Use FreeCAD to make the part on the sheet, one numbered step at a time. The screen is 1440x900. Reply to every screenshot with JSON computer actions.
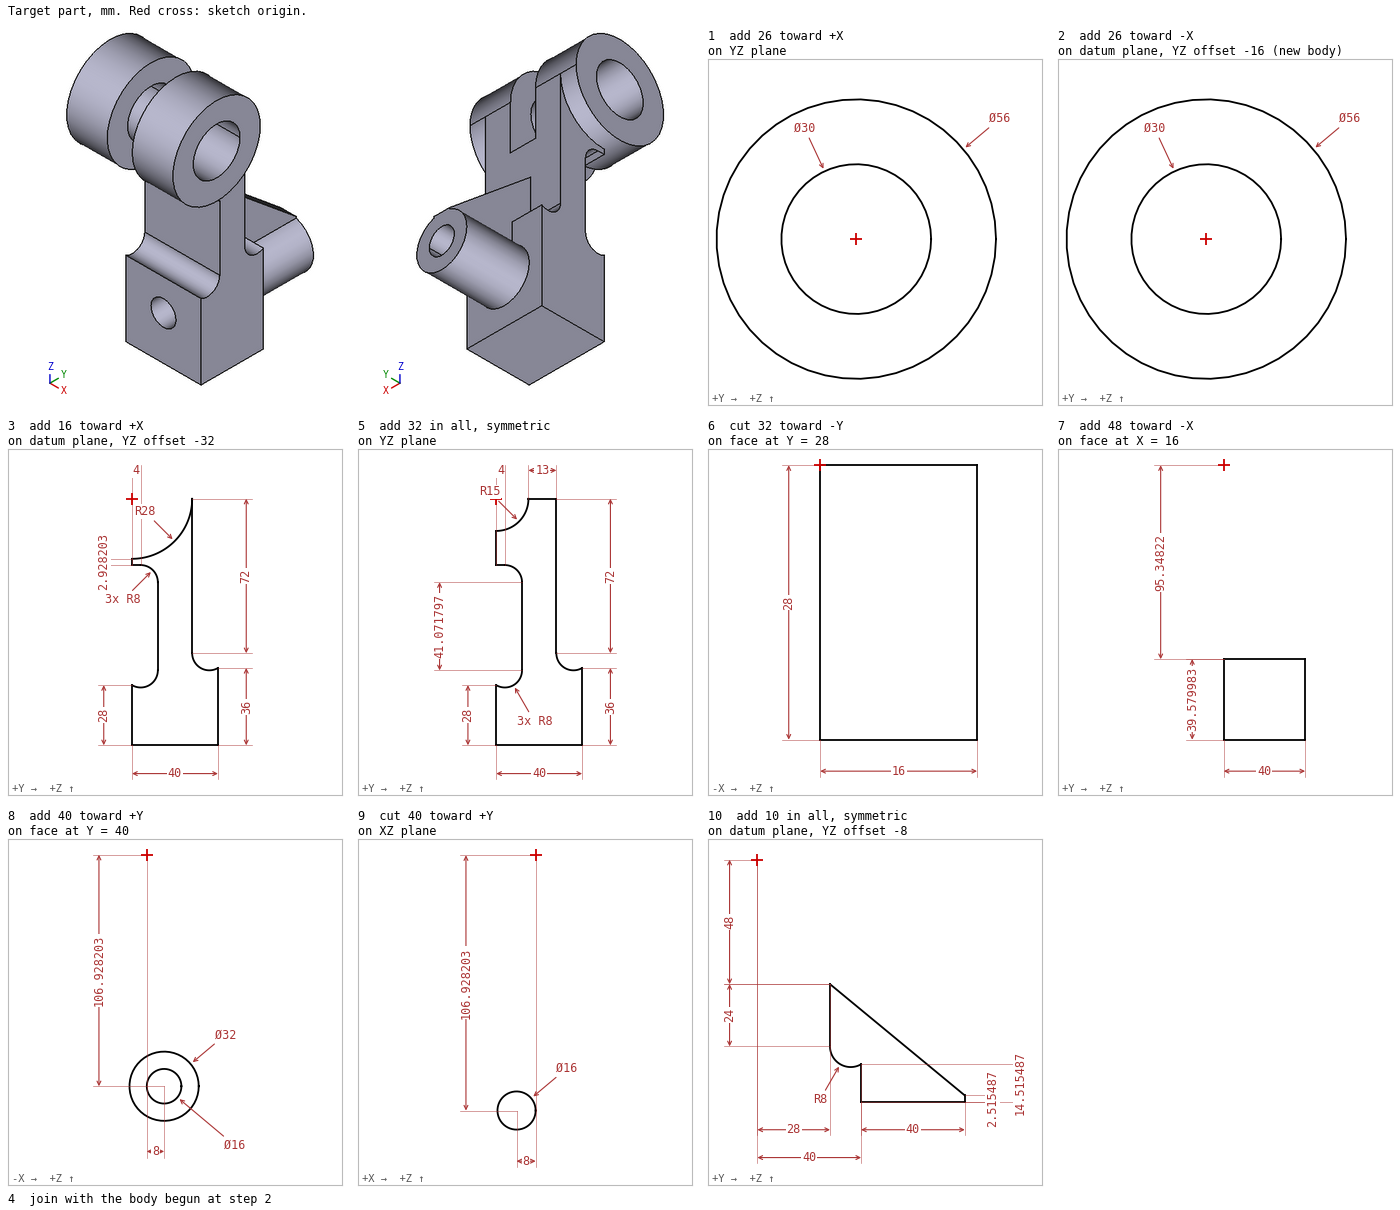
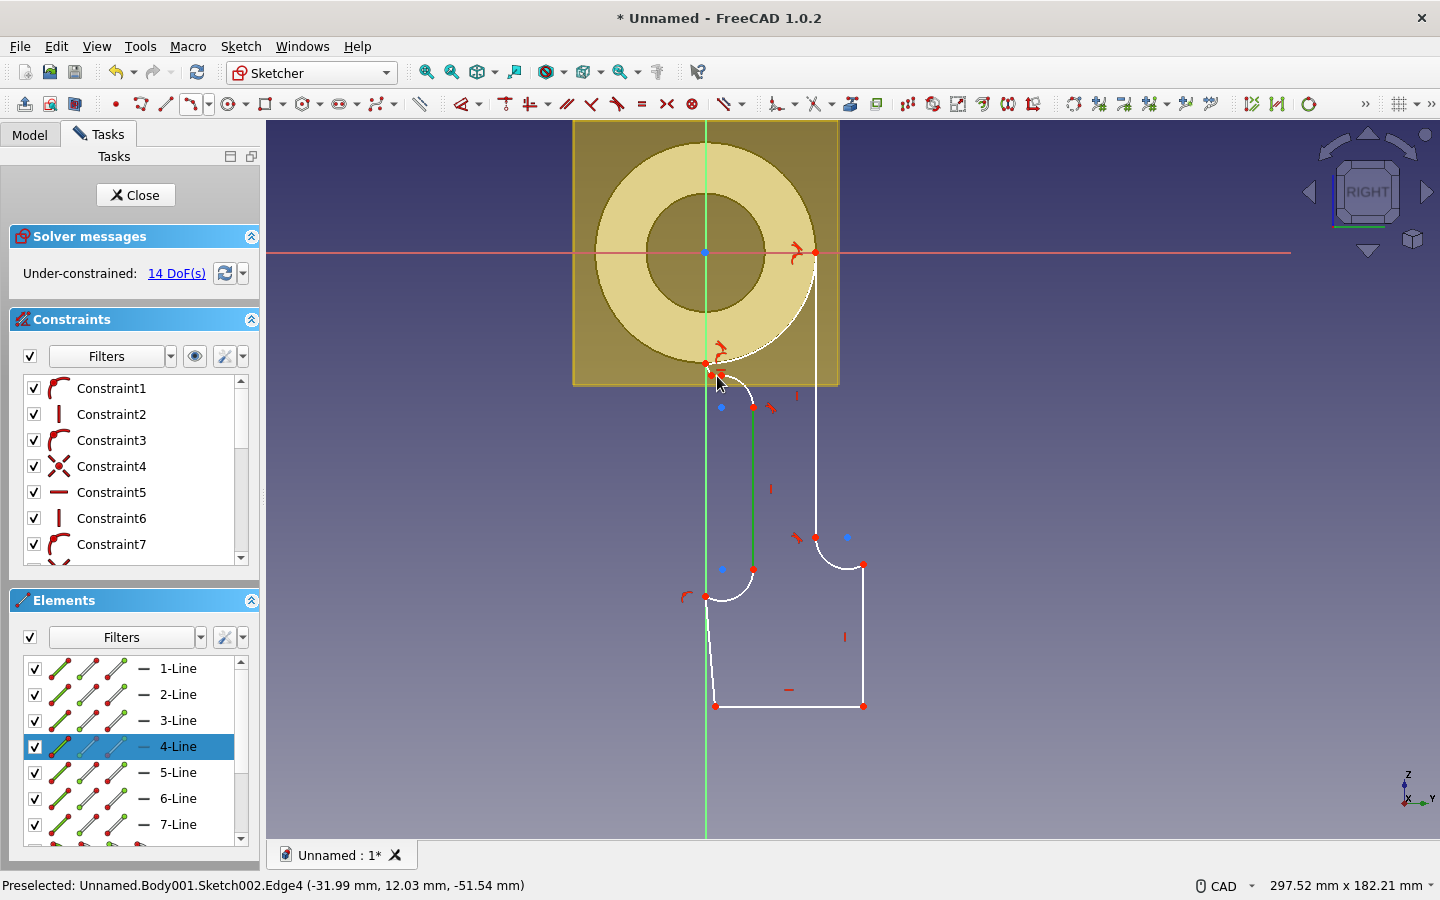
{"action": "left_click", "coordinate": [725, 601]}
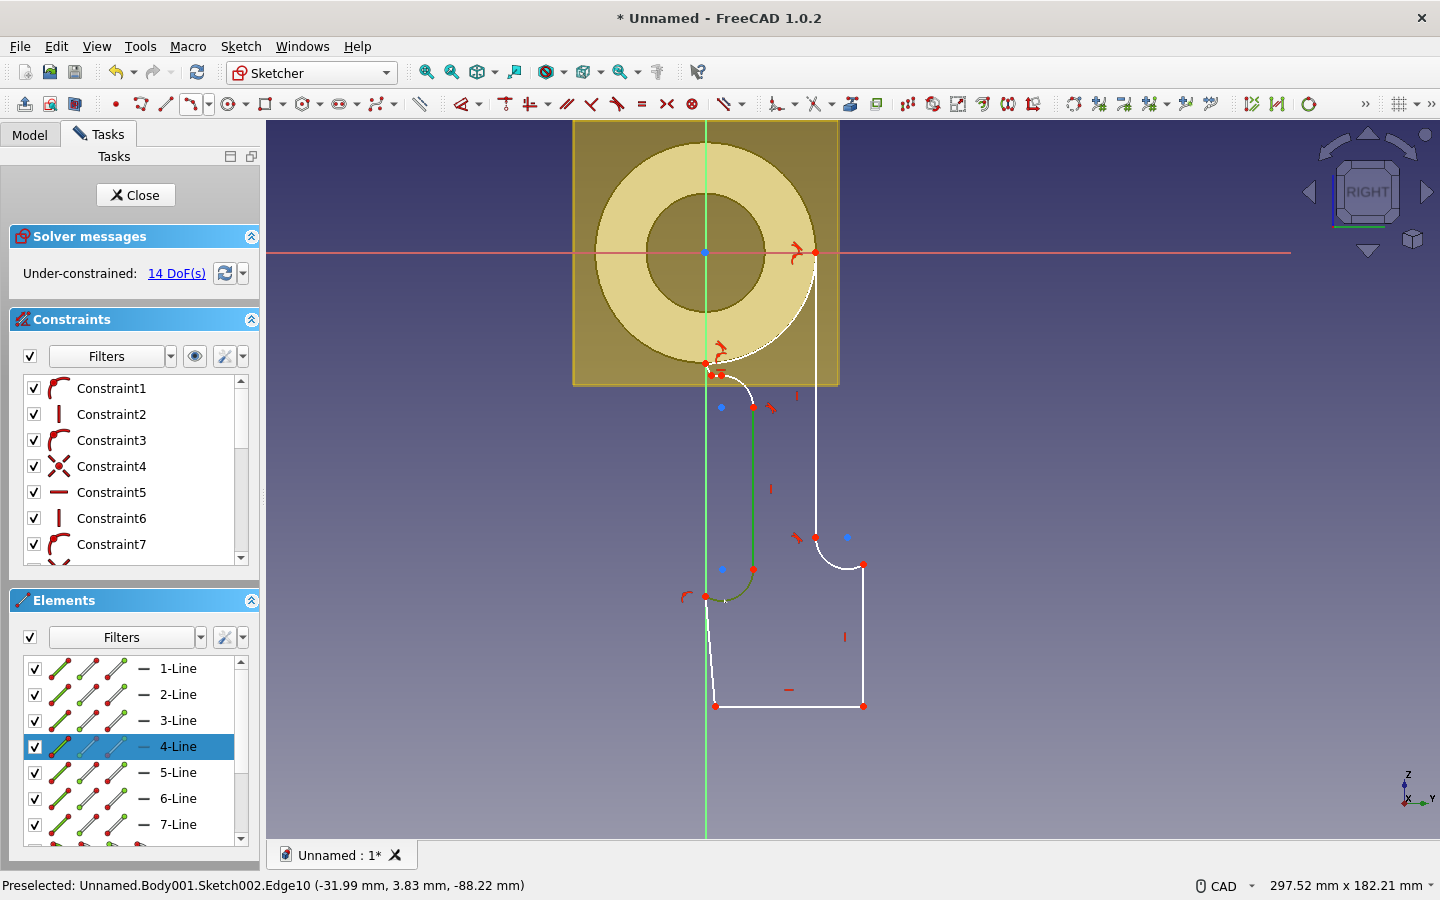
{"action": "left_click", "coordinate": [617, 104]}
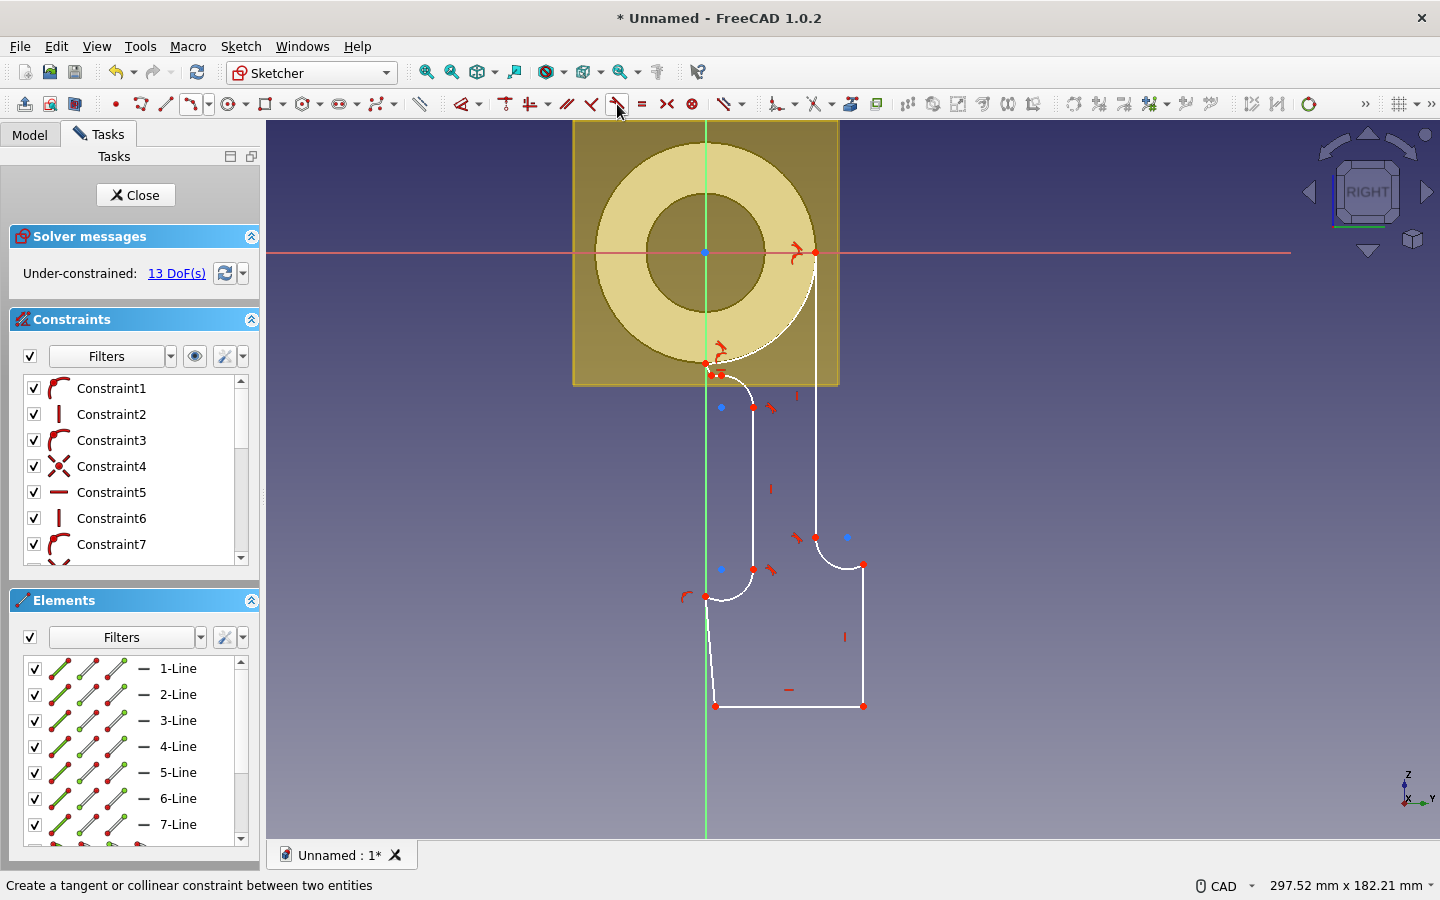
{"action": "scroll", "coordinate": [709, 370], "scroll_direction": "up", "scroll_amount": 5}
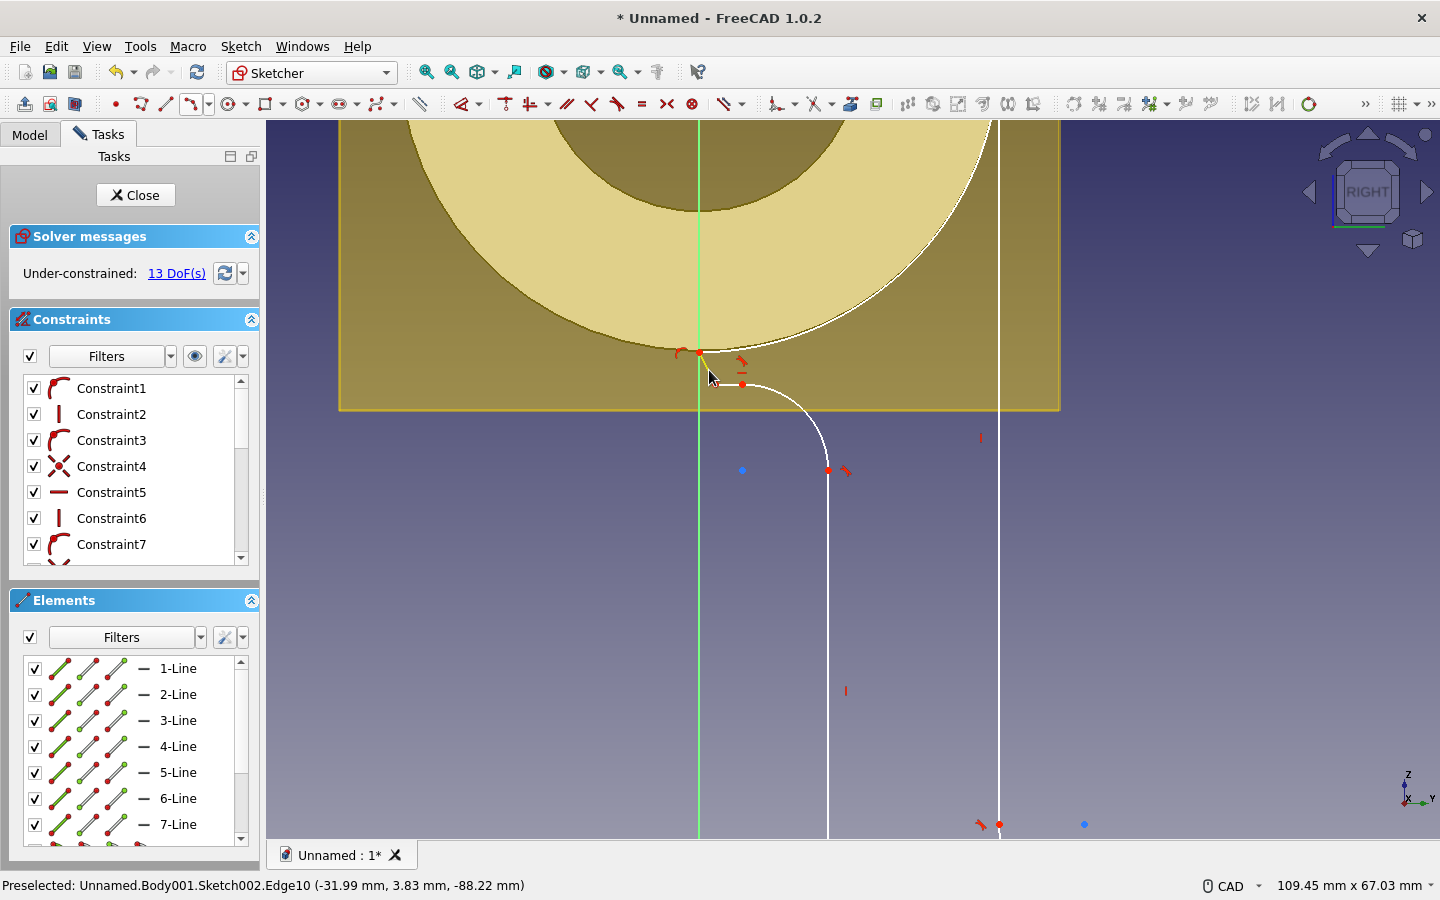
{"action": "left_click", "coordinate": [707, 368]}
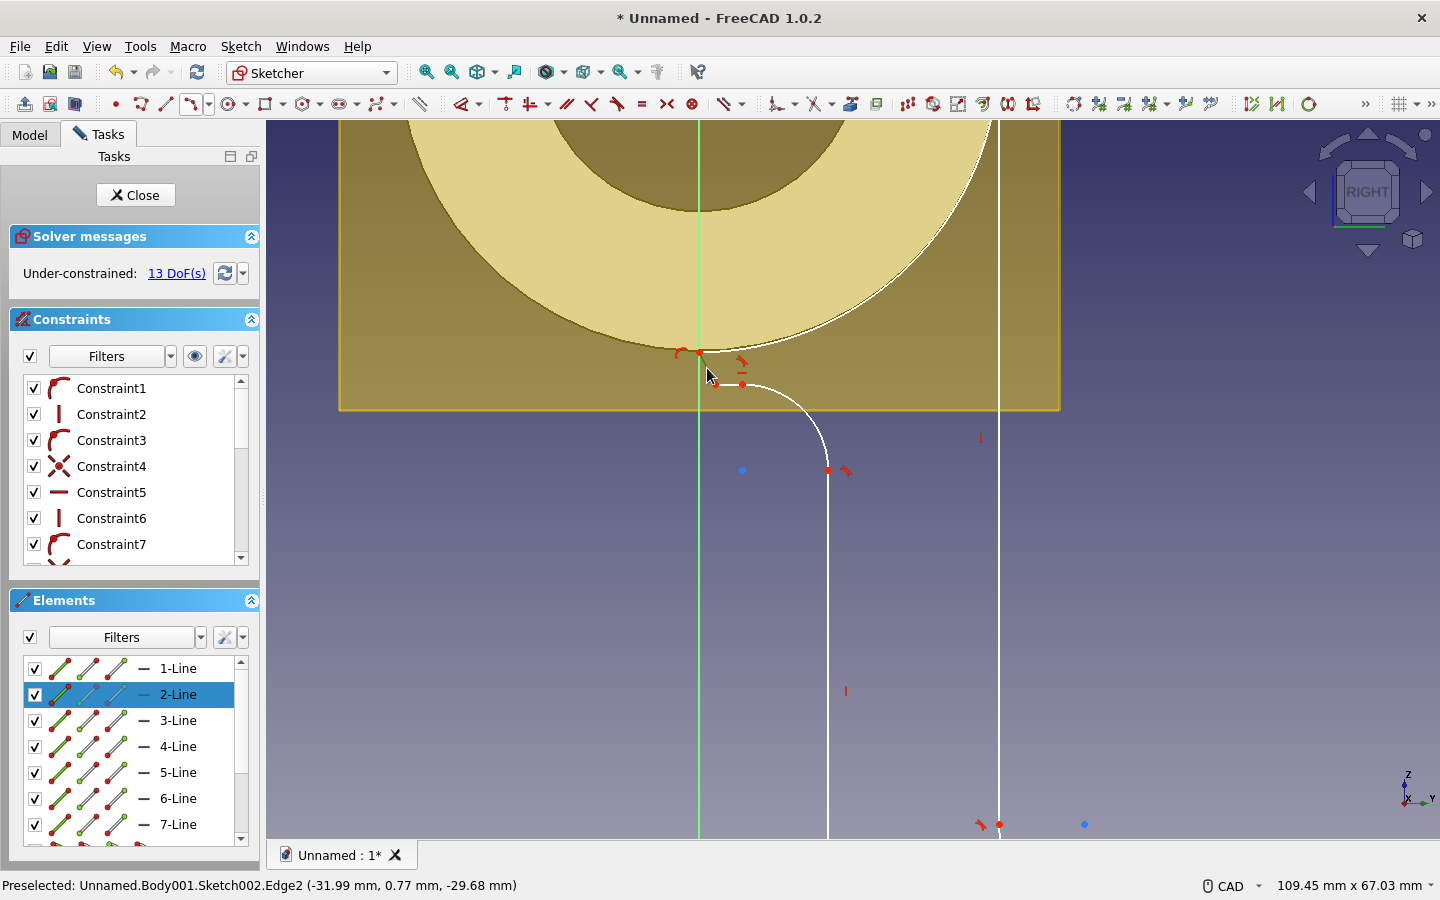
{"action": "key", "text": "v"}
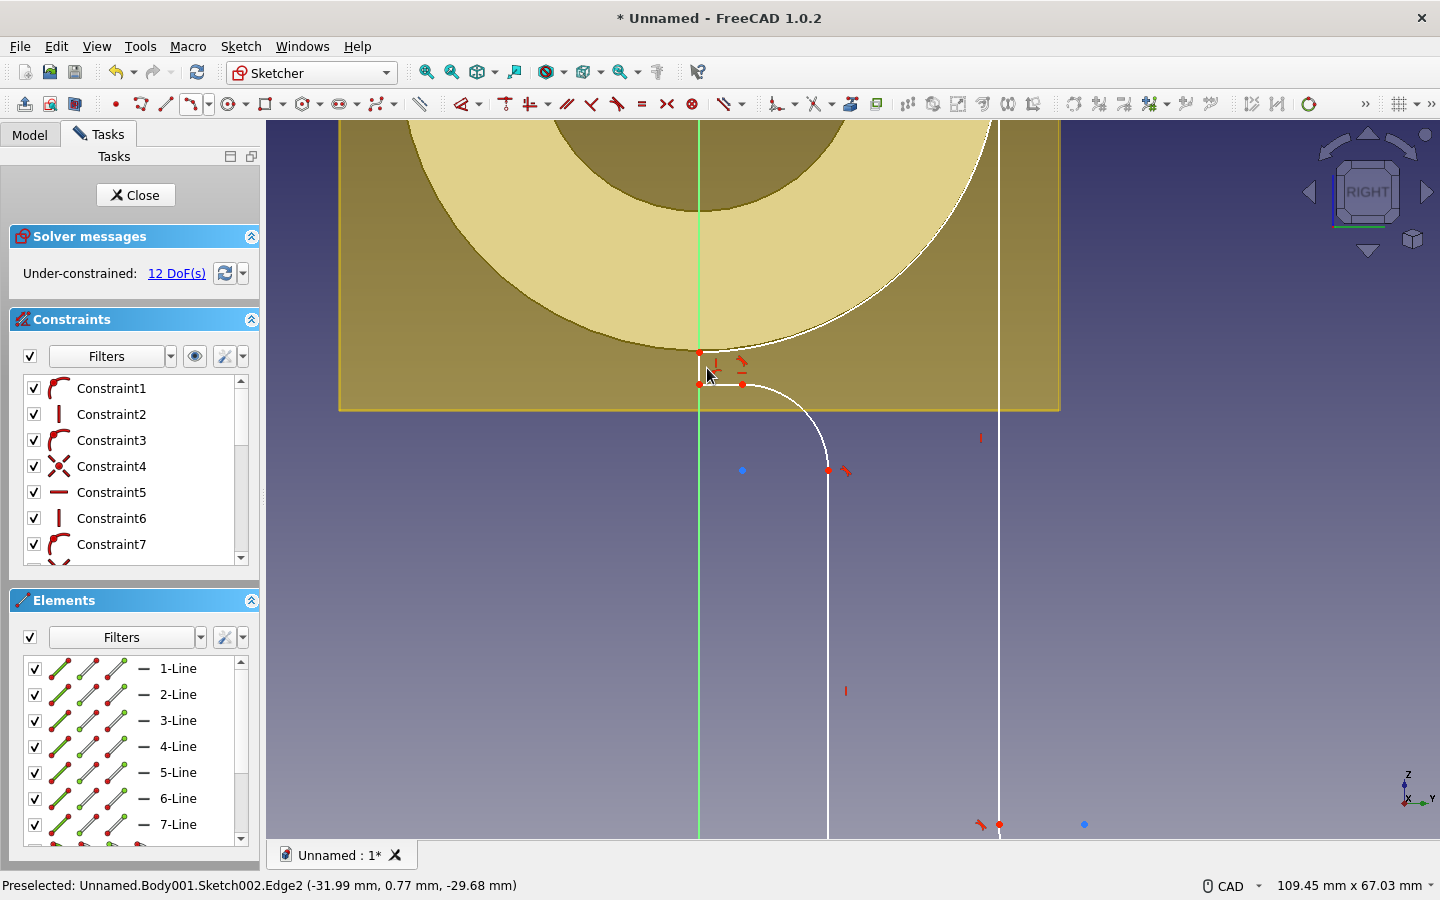
{"action": "scroll", "coordinate": [709, 370], "scroll_direction": "down", "scroll_amount": 5}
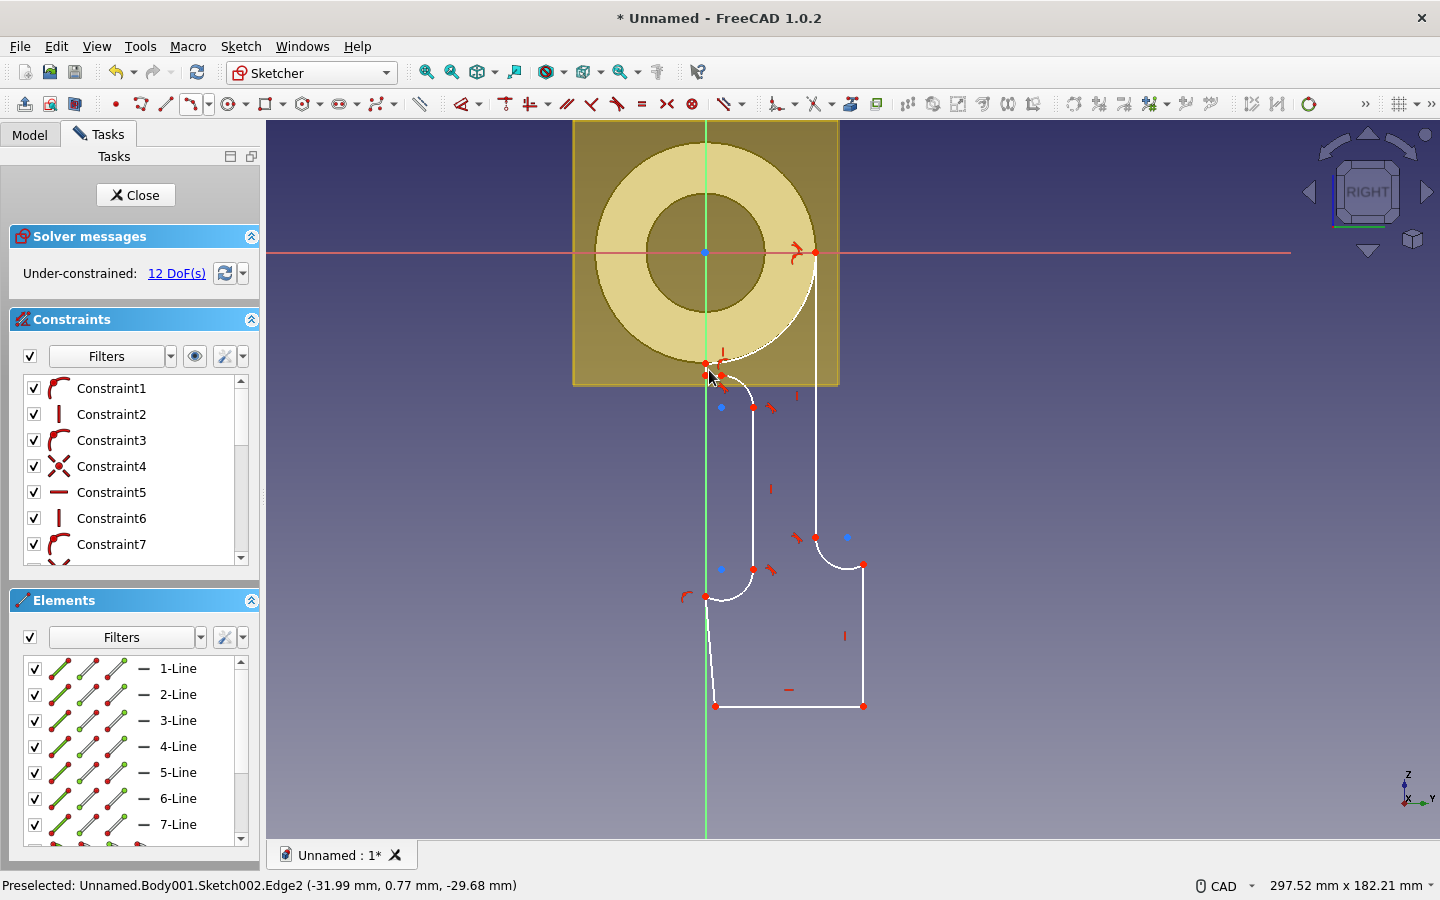
{"action": "scroll", "coordinate": [712, 674], "scroll_direction": "up", "scroll_amount": 4}